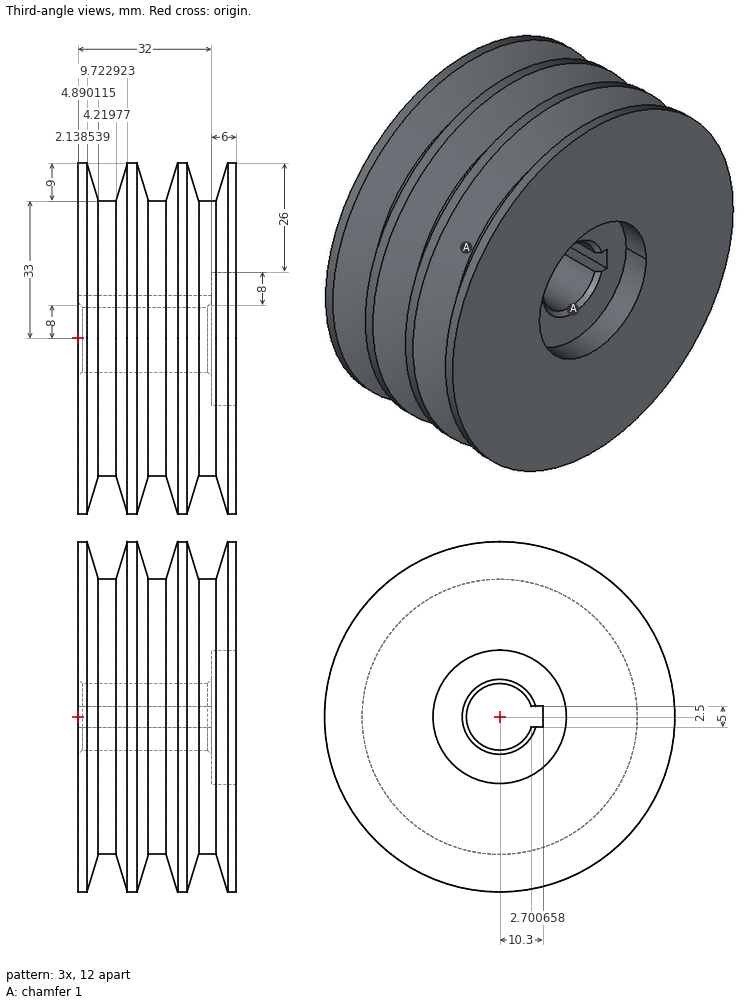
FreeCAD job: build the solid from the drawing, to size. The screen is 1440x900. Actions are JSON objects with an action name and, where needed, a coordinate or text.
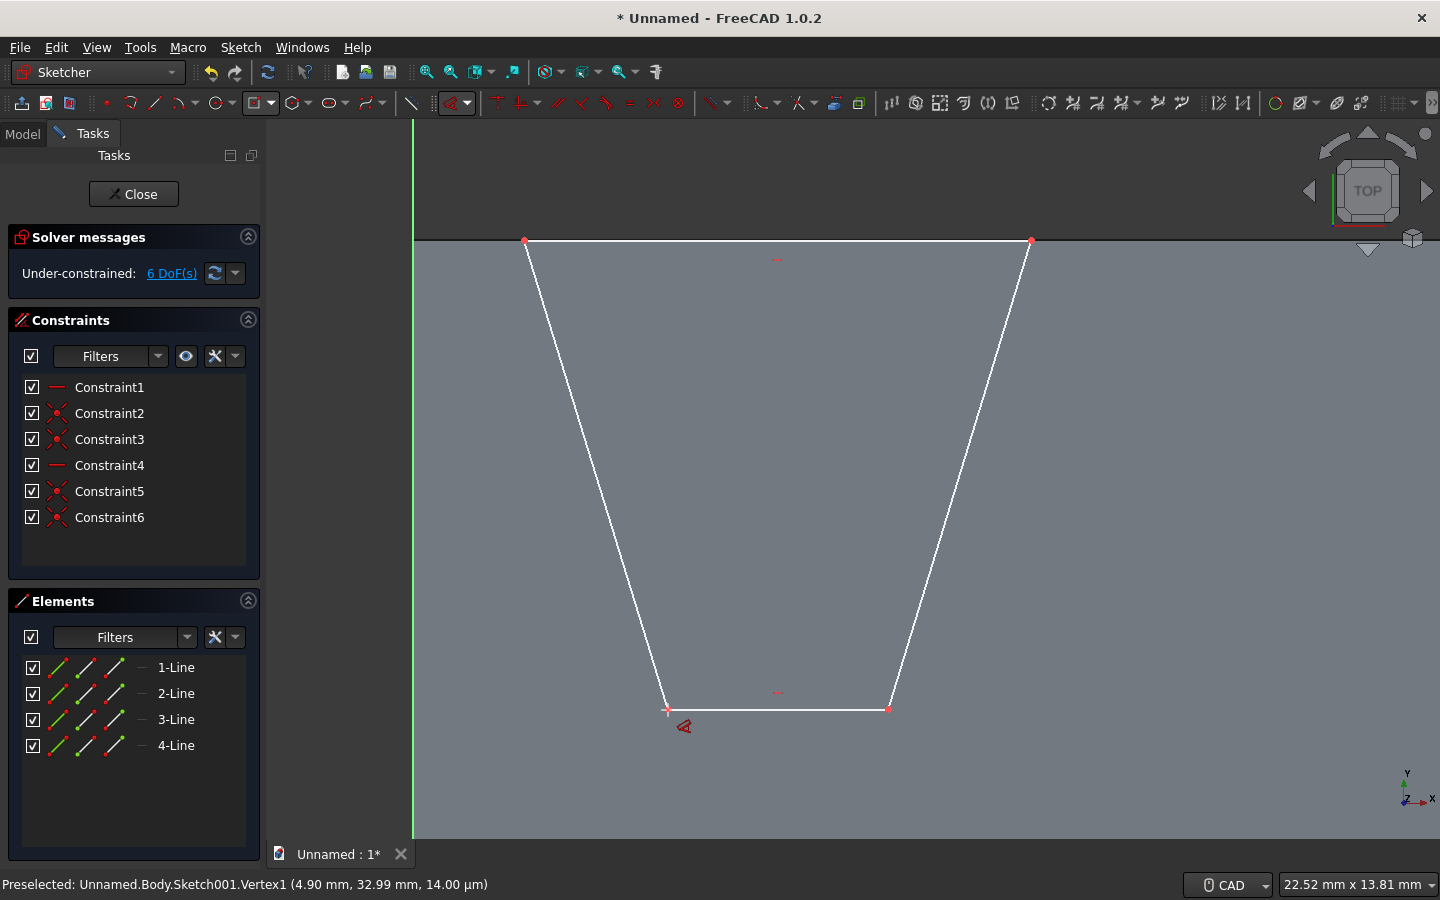
{"action": "left_click", "coordinate": [931, 569]}
{"action": "left_click", "coordinate": [1065, 476]}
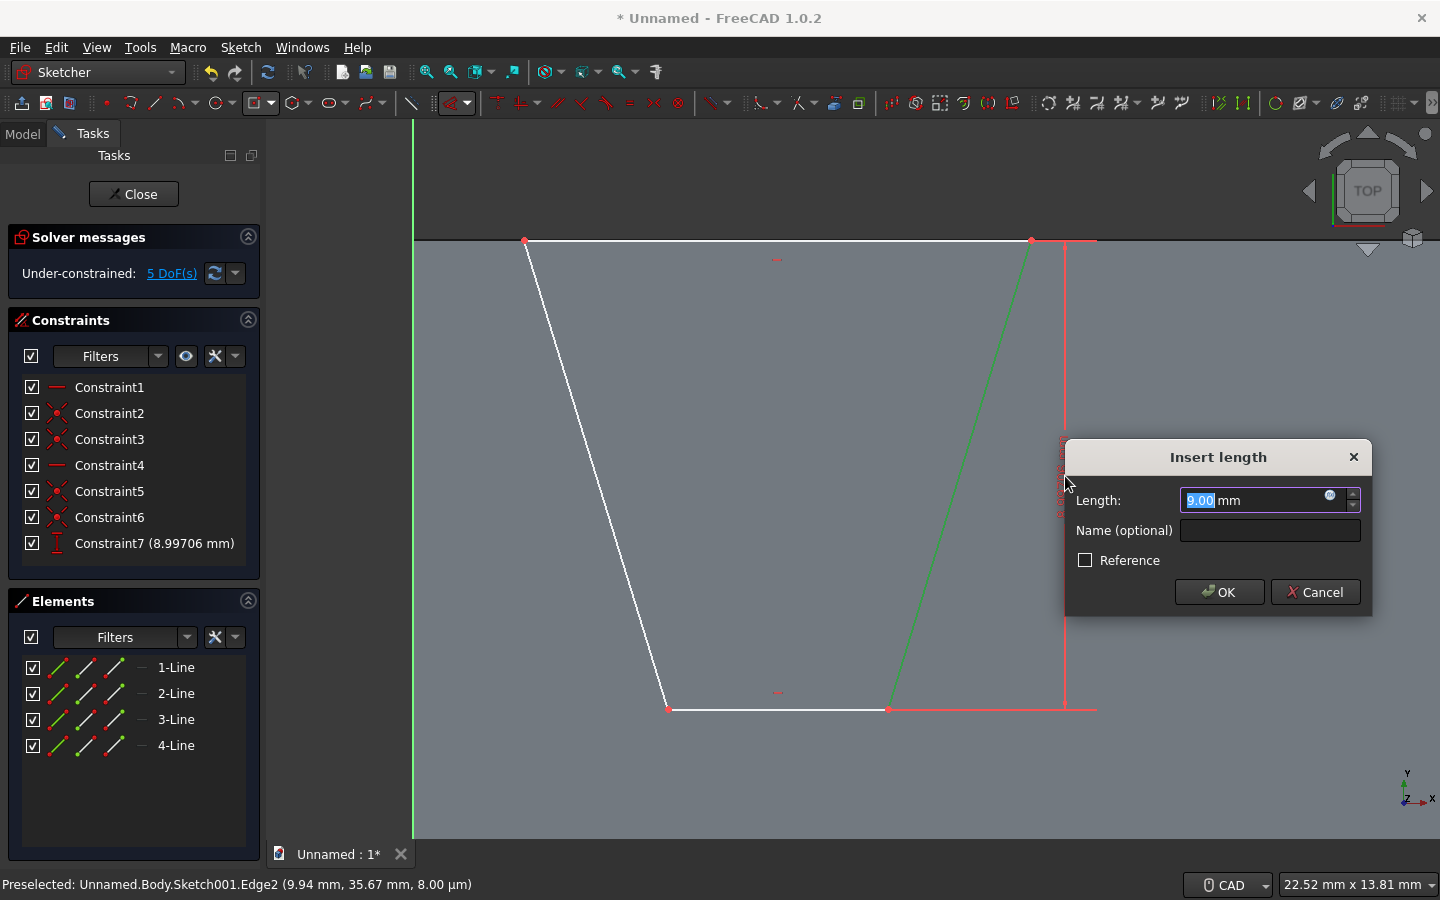
{"action": "type", "text": "9"}
{"action": "key", "text": "Return"}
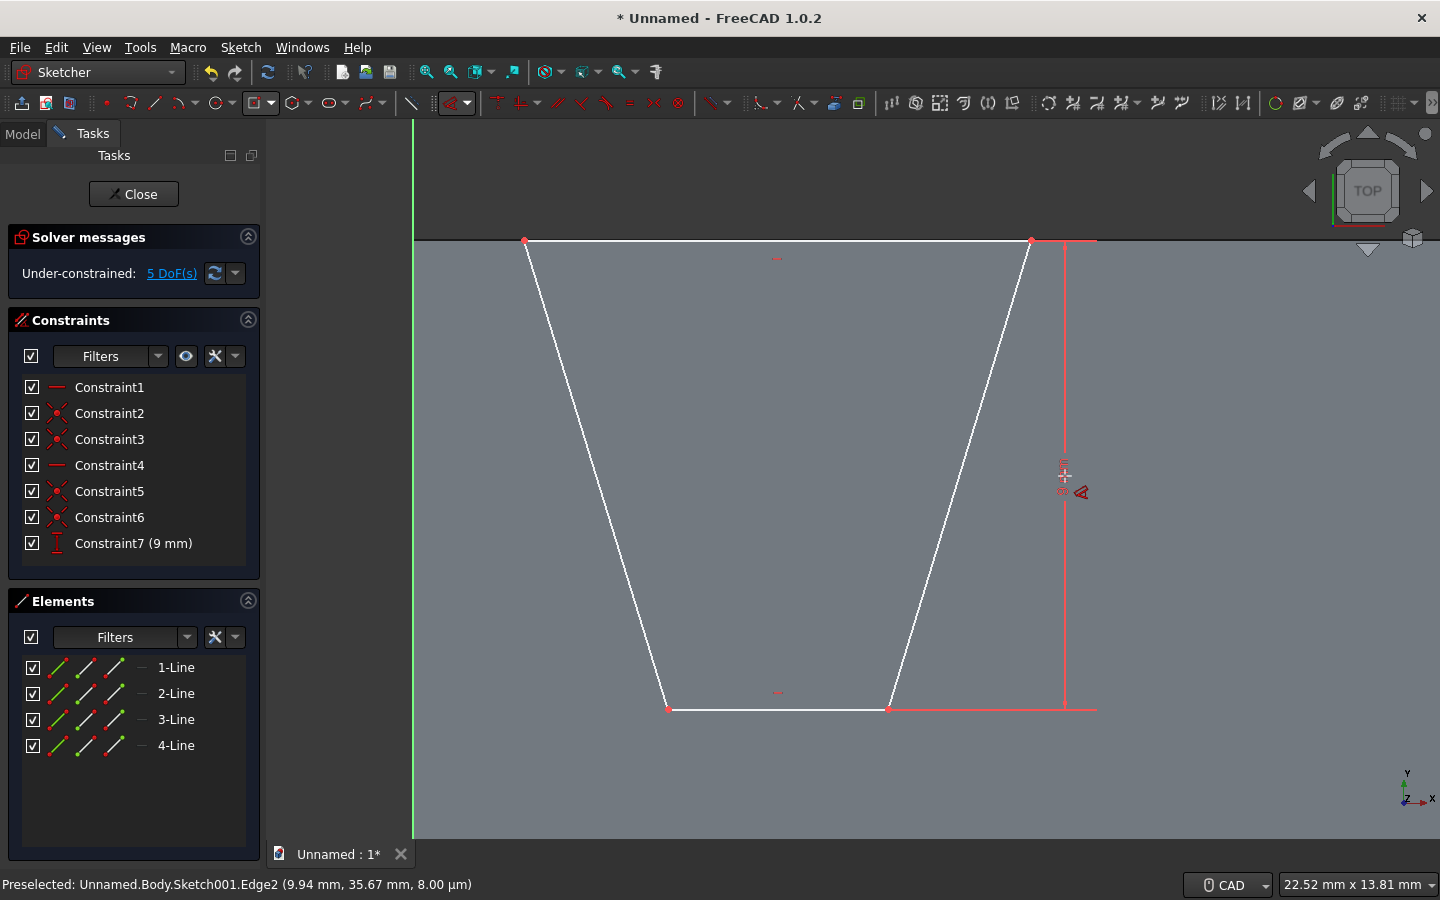
{"action": "left_click", "coordinate": [668, 710]}
{"action": "left_click", "coordinate": [379, 761]}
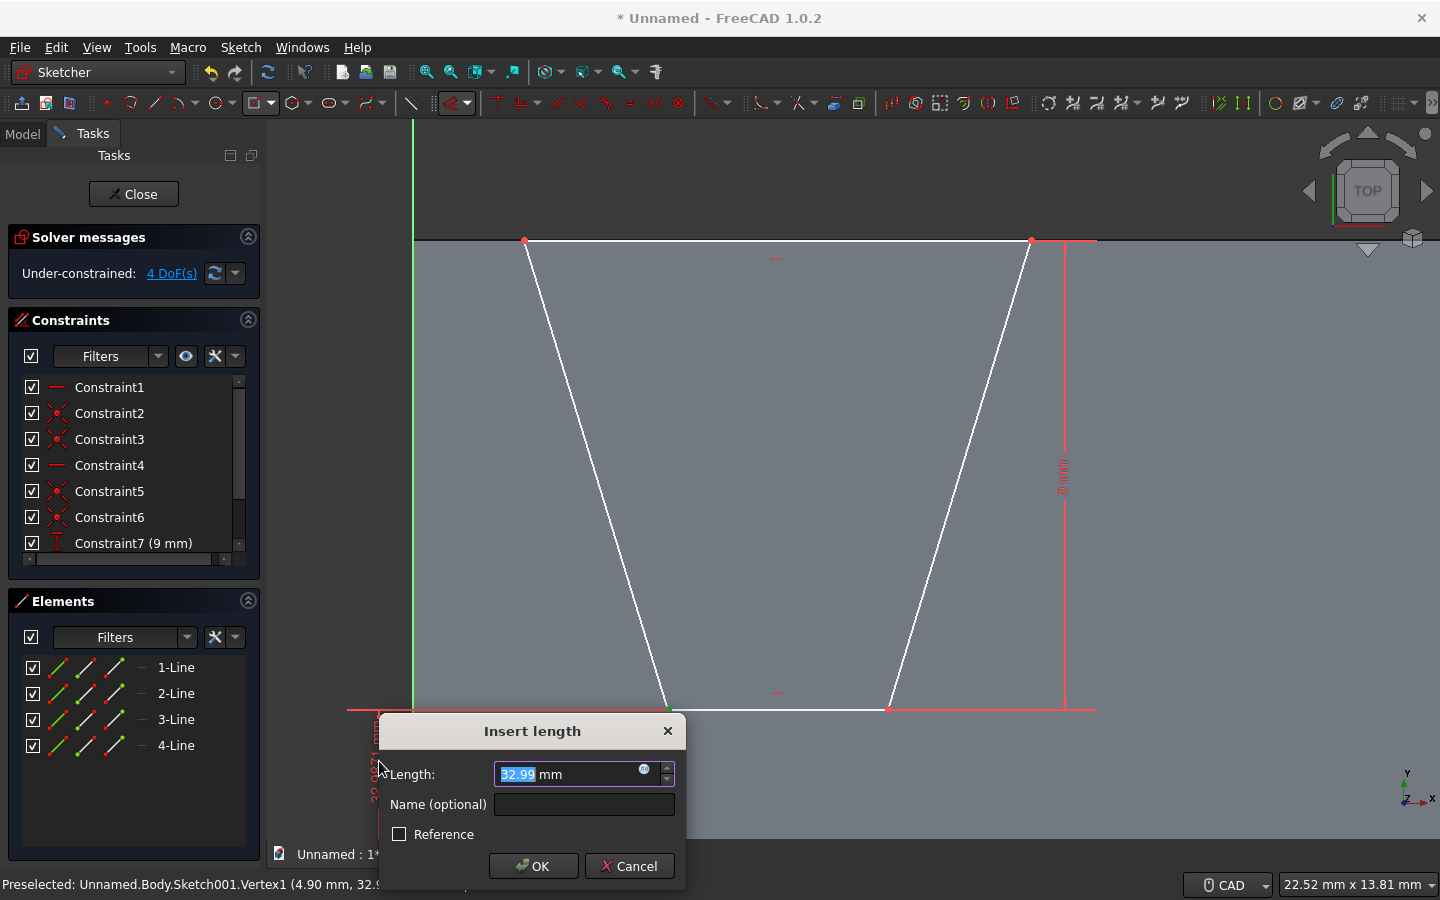
{"action": "type", "text": "33"}
{"action": "key", "text": "Return"}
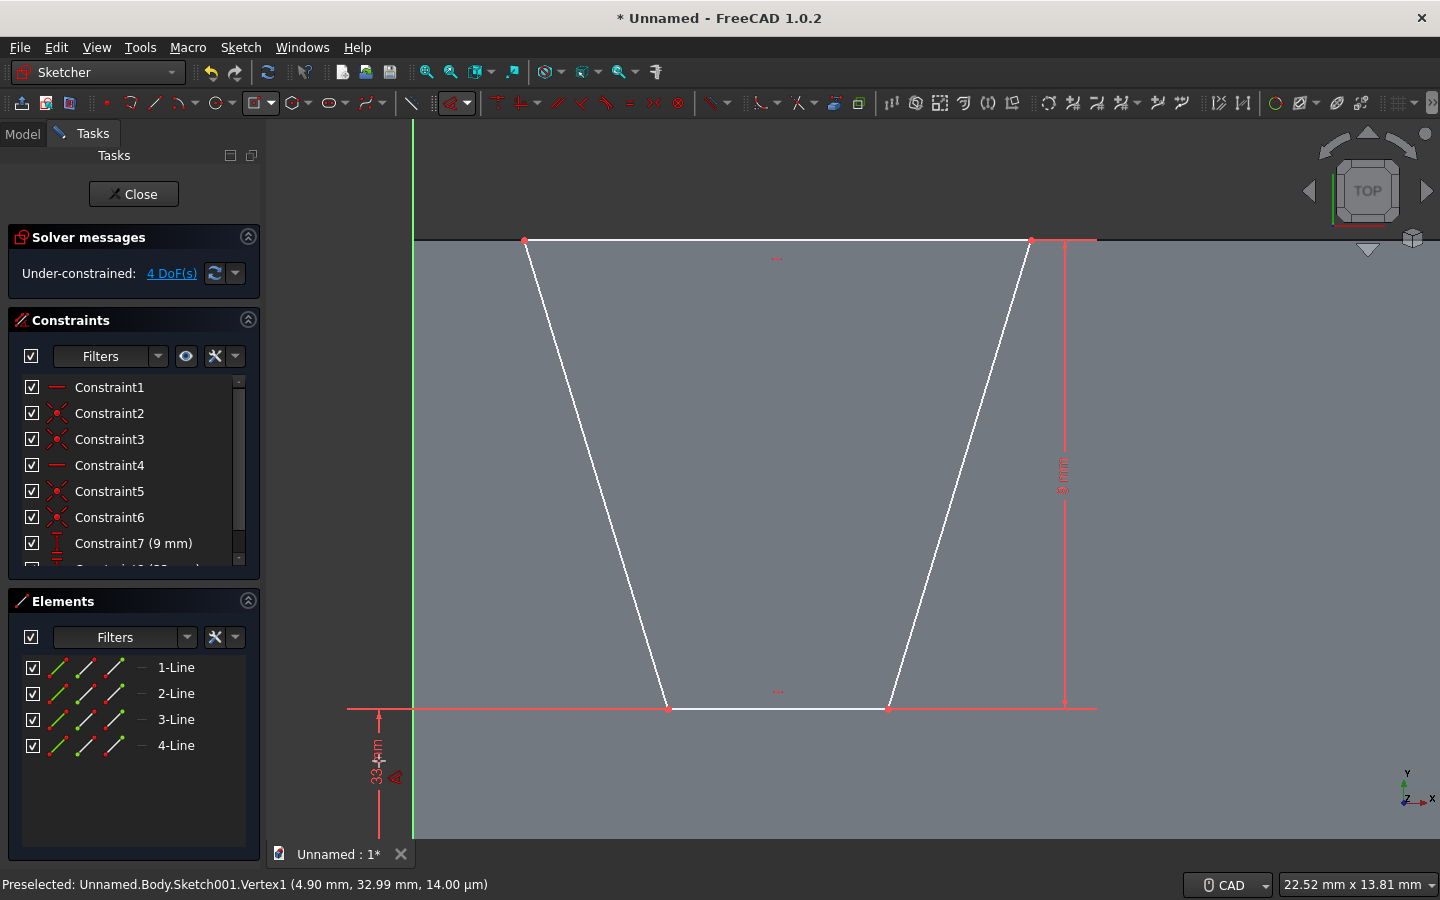
{"action": "left_click", "coordinate": [734, 709]}
{"action": "left_click", "coordinate": [778, 743]}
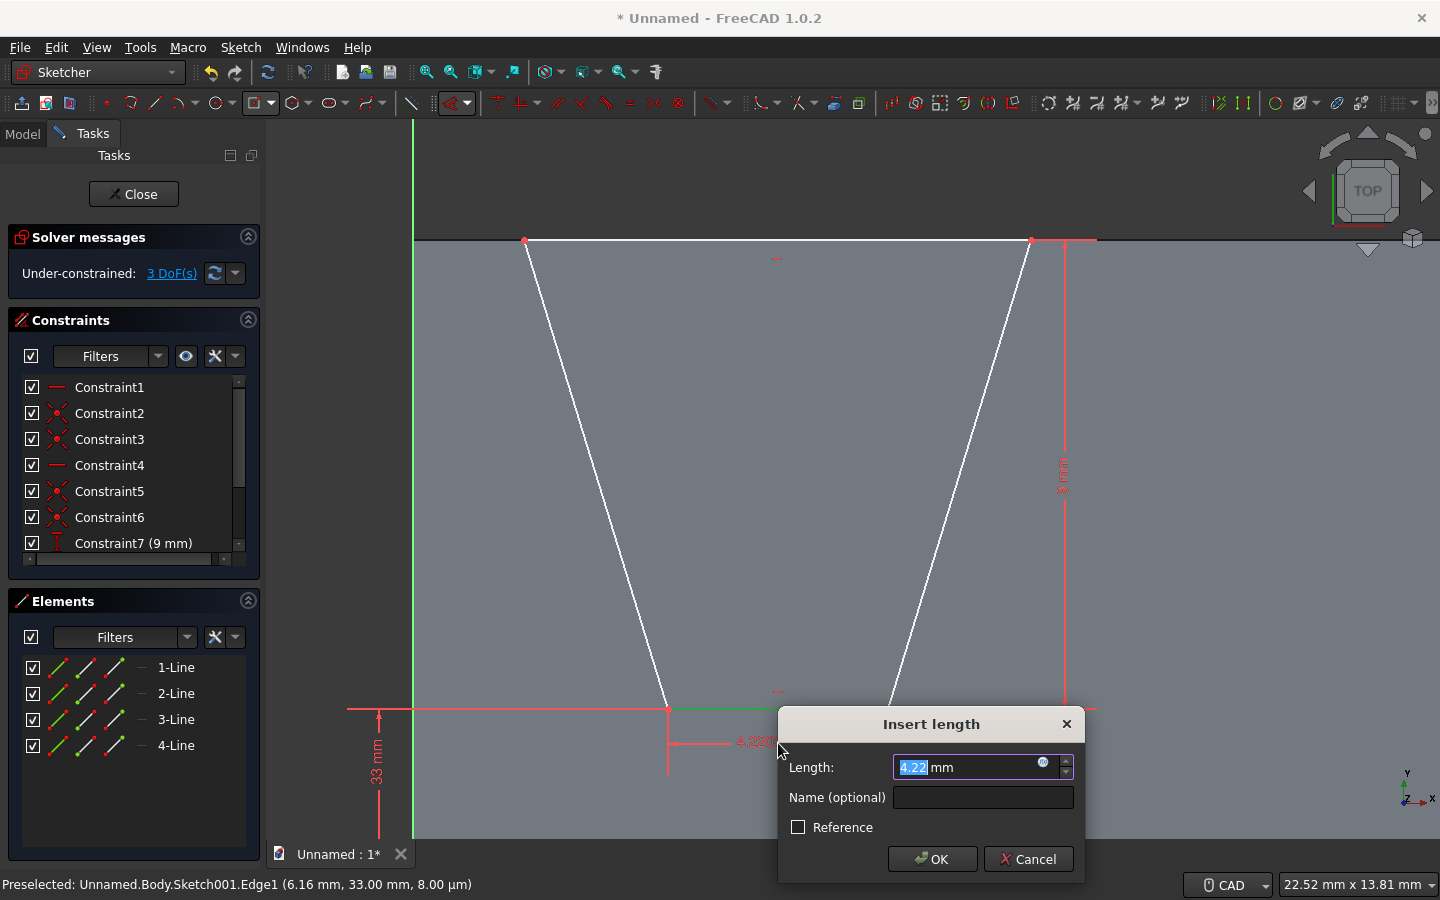
{"action": "type", "text": "4.21977"}
{"action": "key", "text": "Return"}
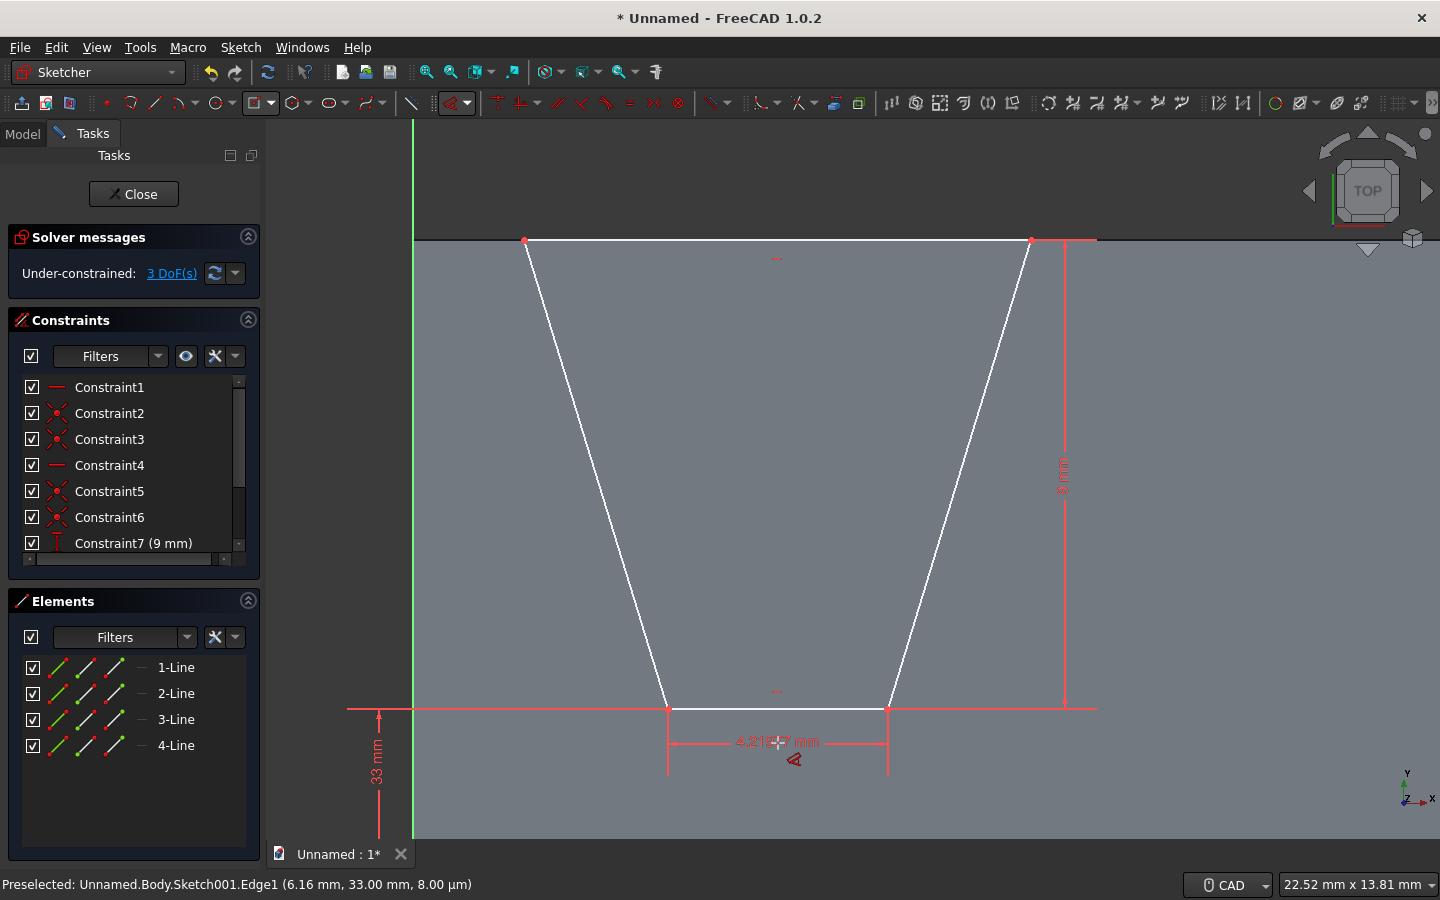
{"action": "left_click", "coordinate": [879, 240]}
{"action": "left_click", "coordinate": [777, 206]}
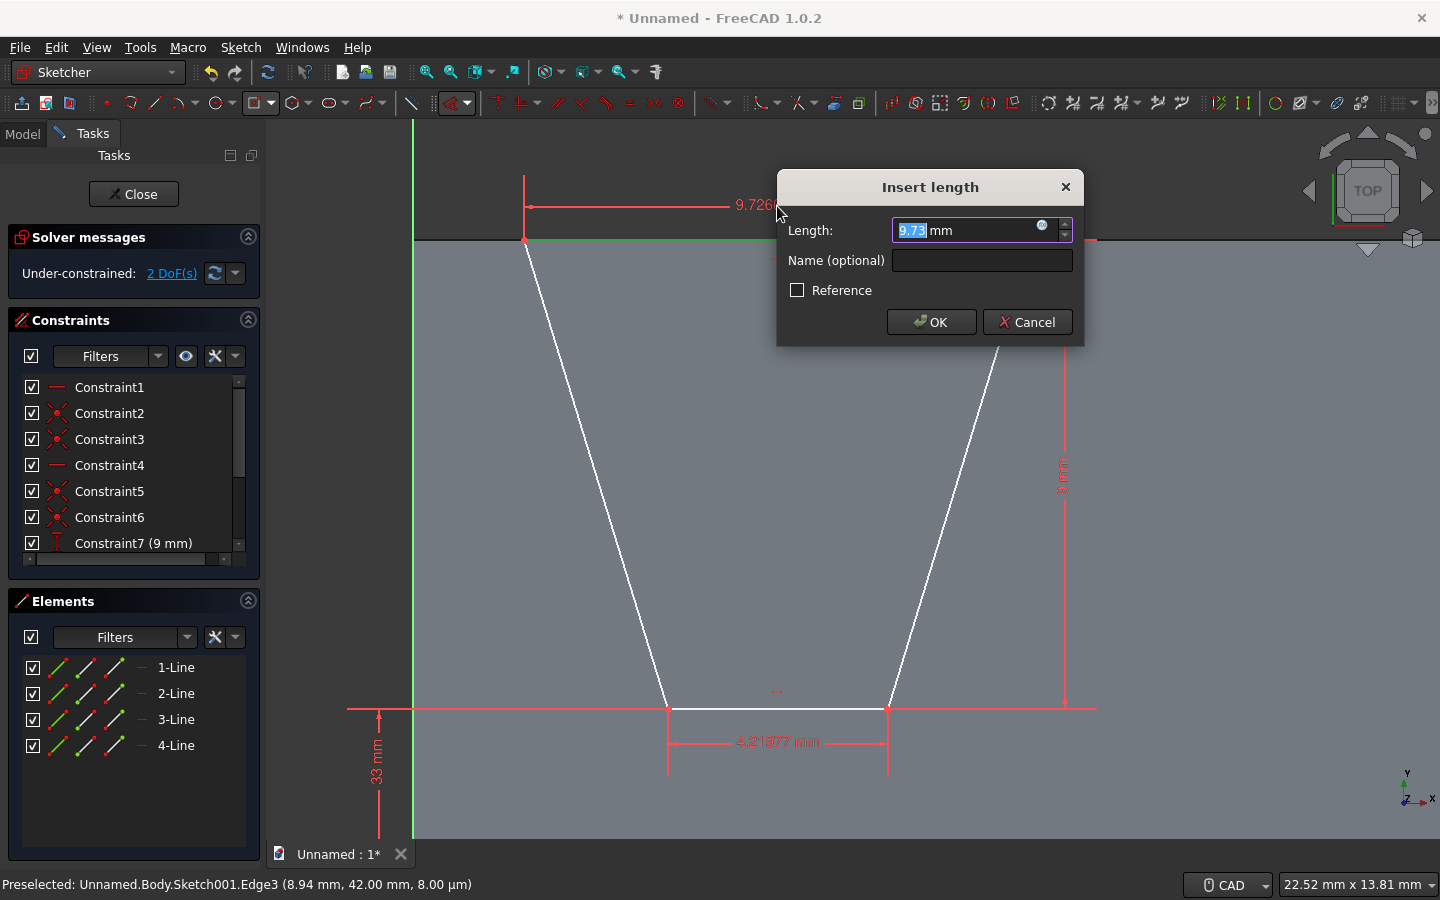
{"action": "type", "text": "9.722923"}
{"action": "key", "text": "Return"}